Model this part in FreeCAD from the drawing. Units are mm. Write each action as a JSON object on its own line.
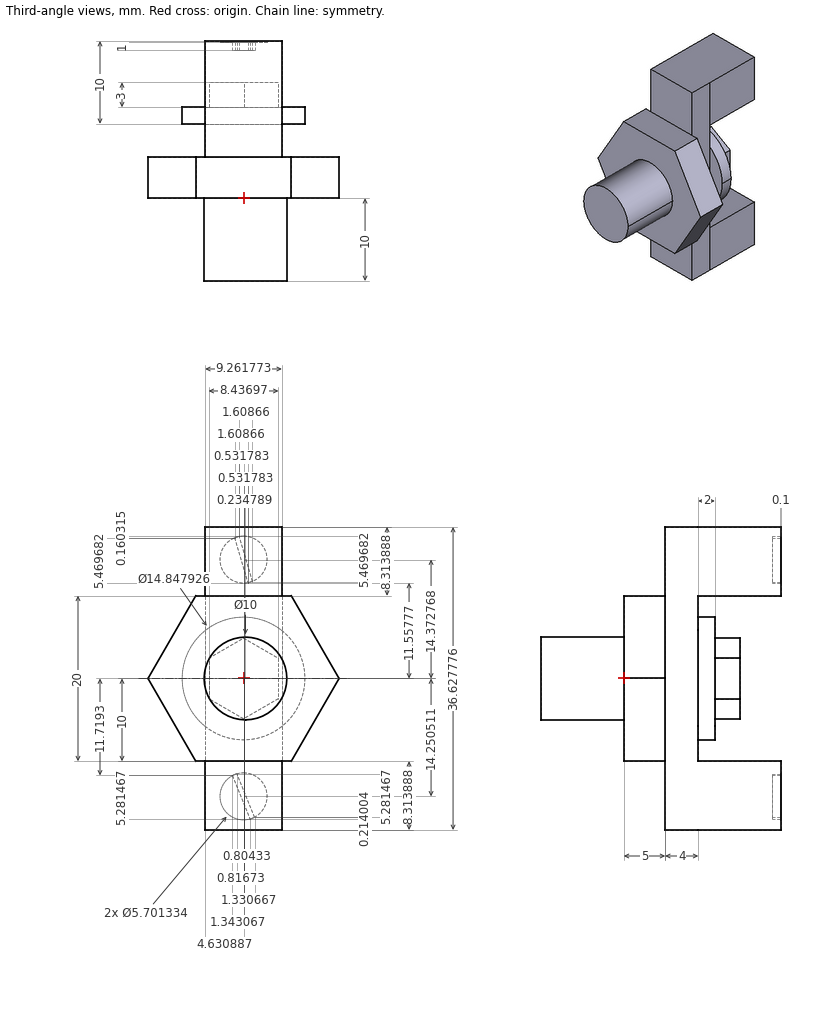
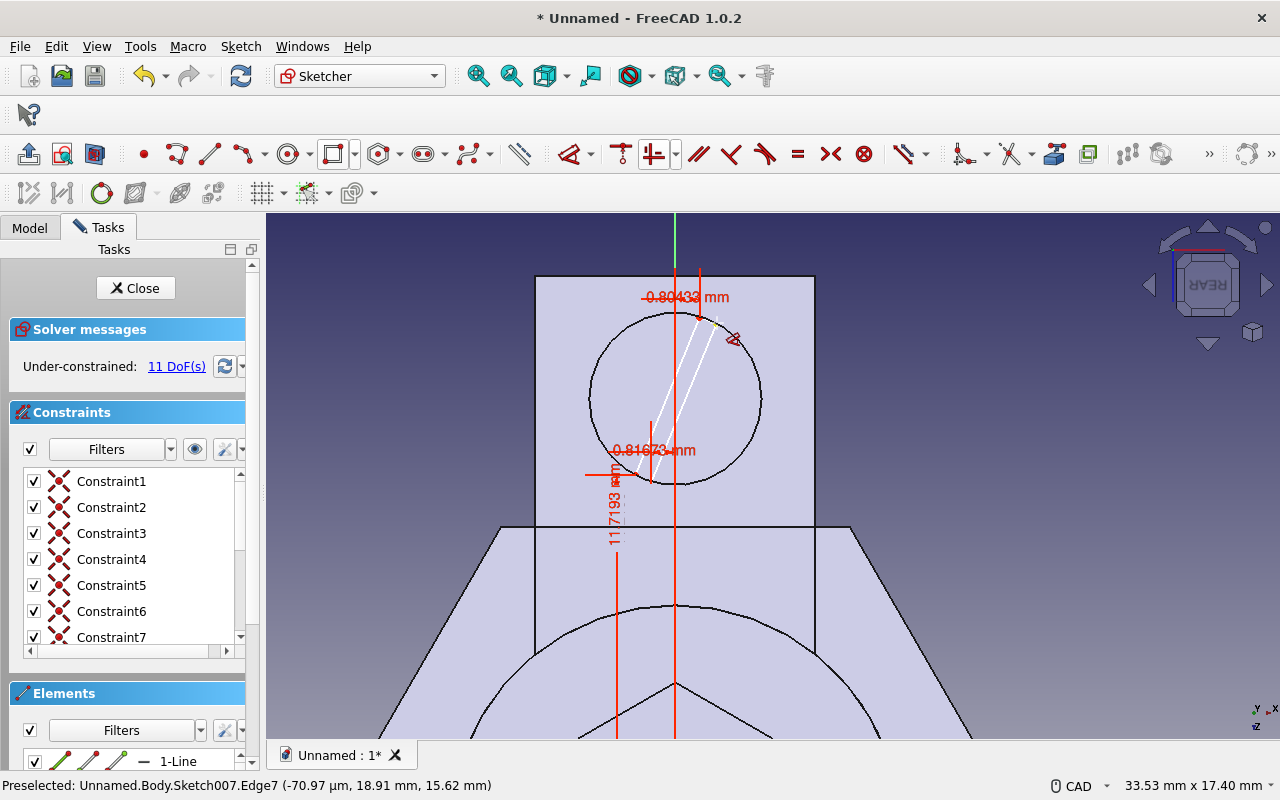
{"action": "left_click", "coordinate": [717, 324]}
{"action": "left_click", "coordinate": [696, 266]}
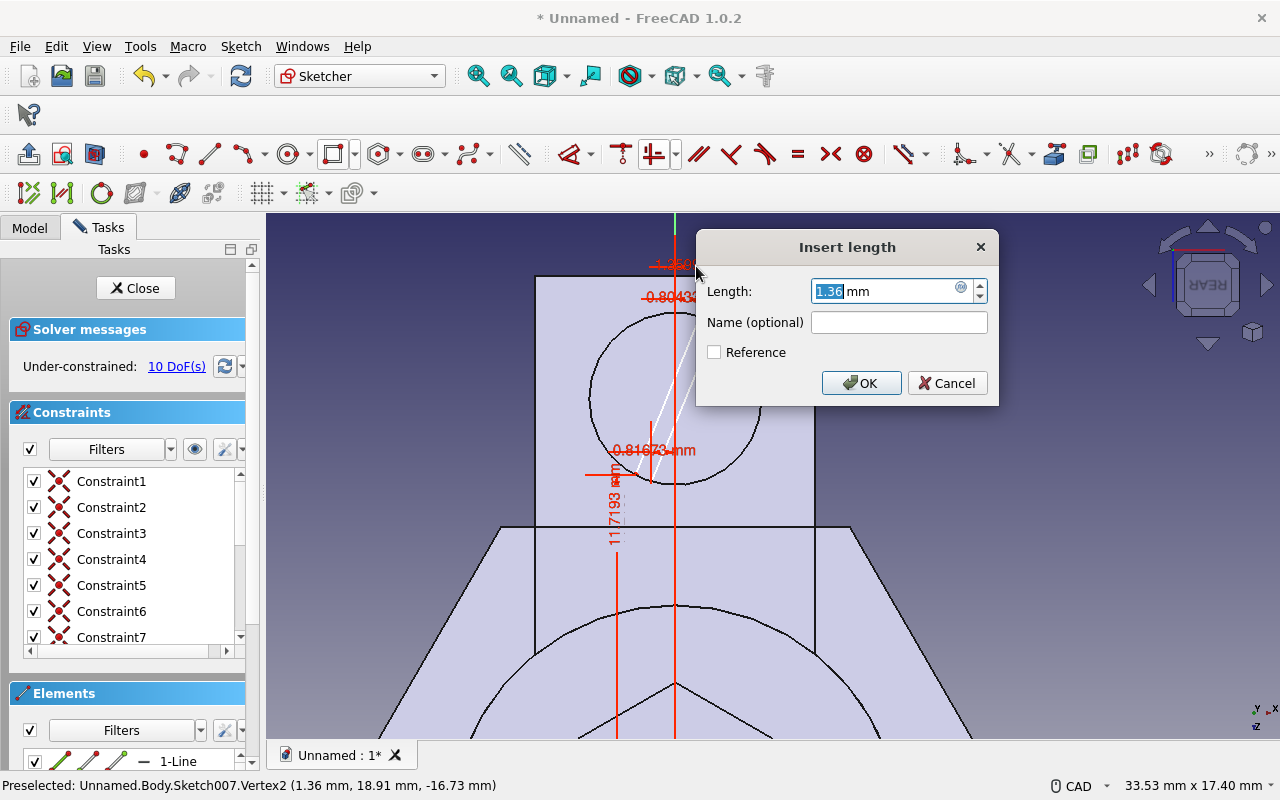
{"action": "type", "text": "1.330667"}
{"action": "key", "text": "Return"}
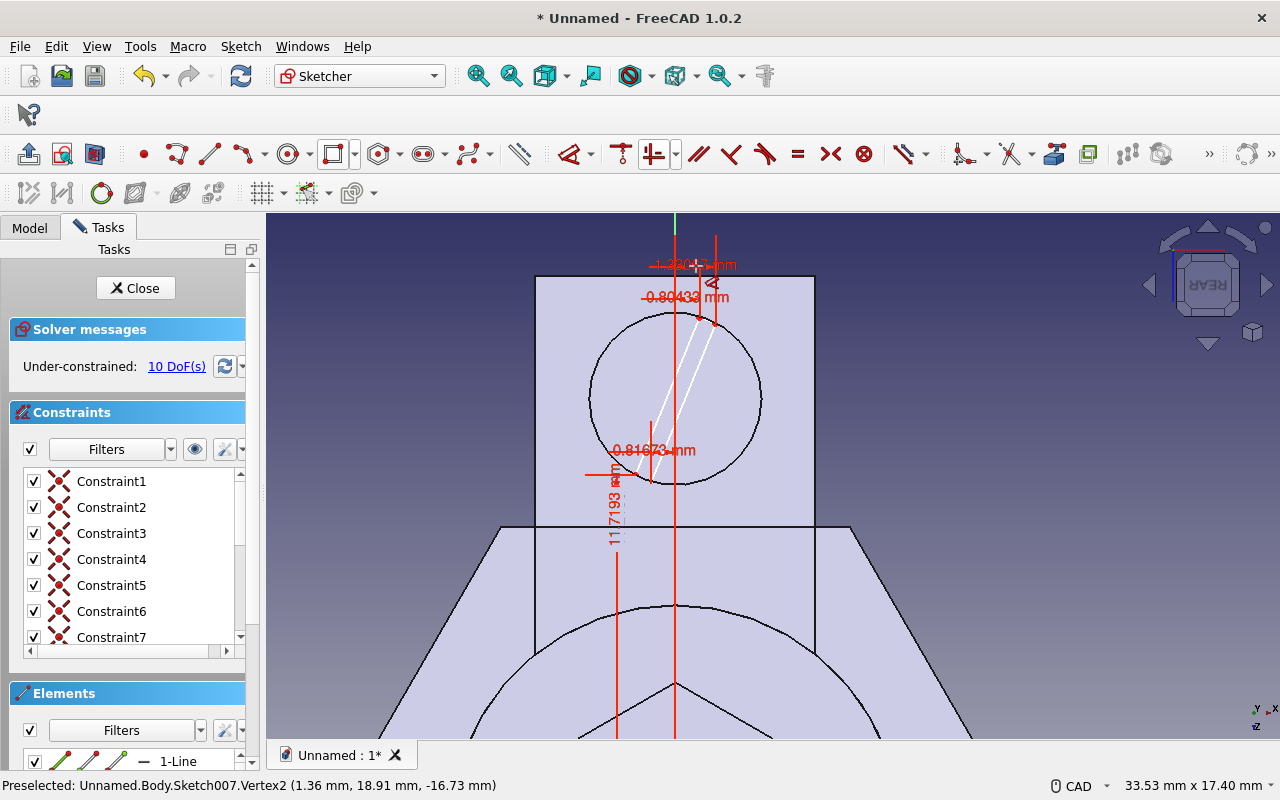
{"action": "left_click", "coordinate": [635, 475]}
{"action": "left_click", "coordinate": [641, 417]}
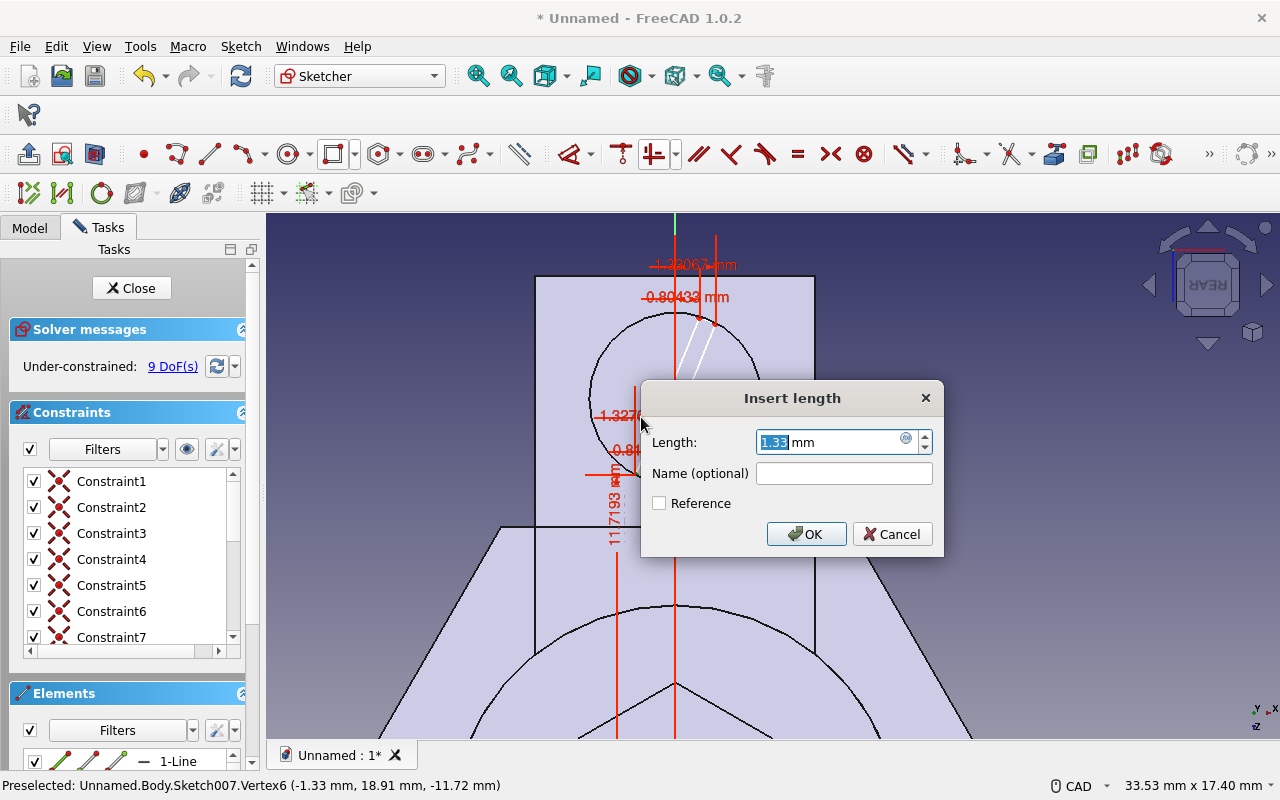
{"action": "type", "text": "1.343067"}
{"action": "key", "text": "Return"}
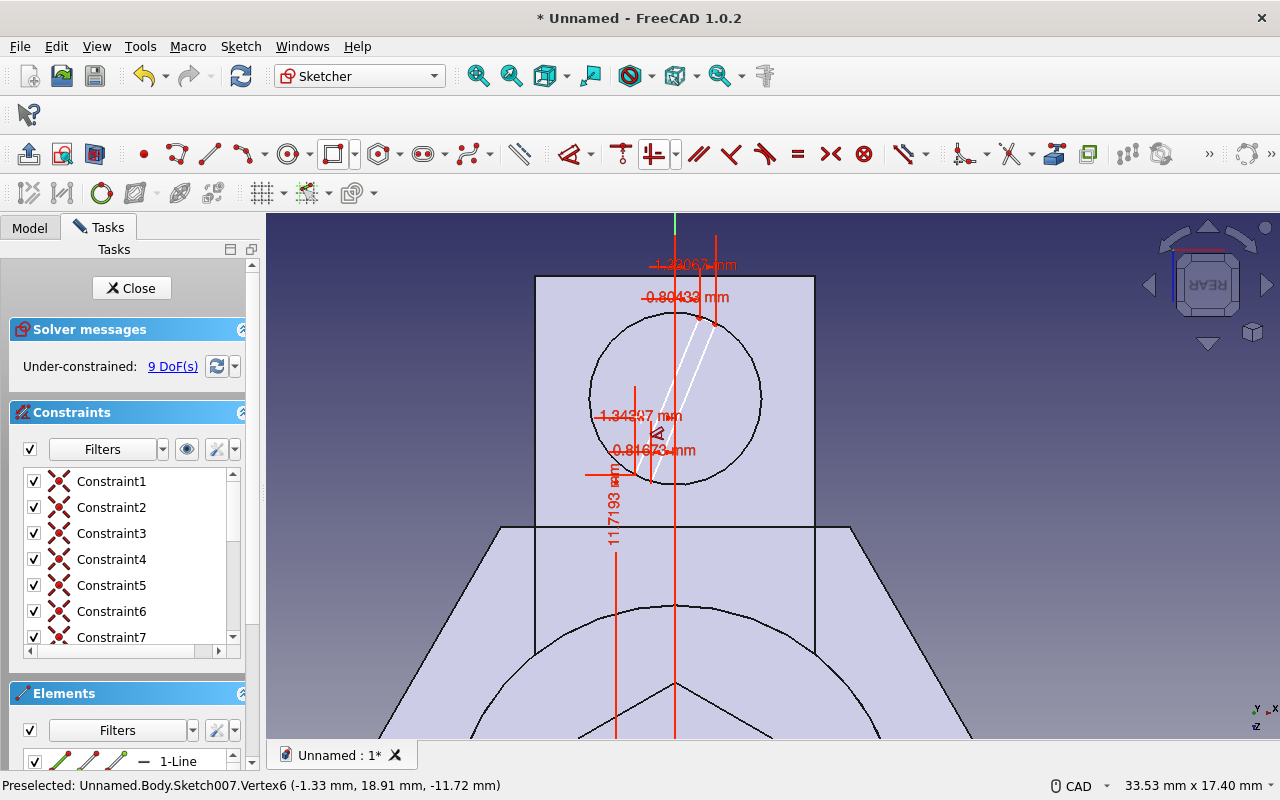
{"action": "scroll", "coordinate": [717, 322], "scroll_direction": "down", "scroll_amount": 6}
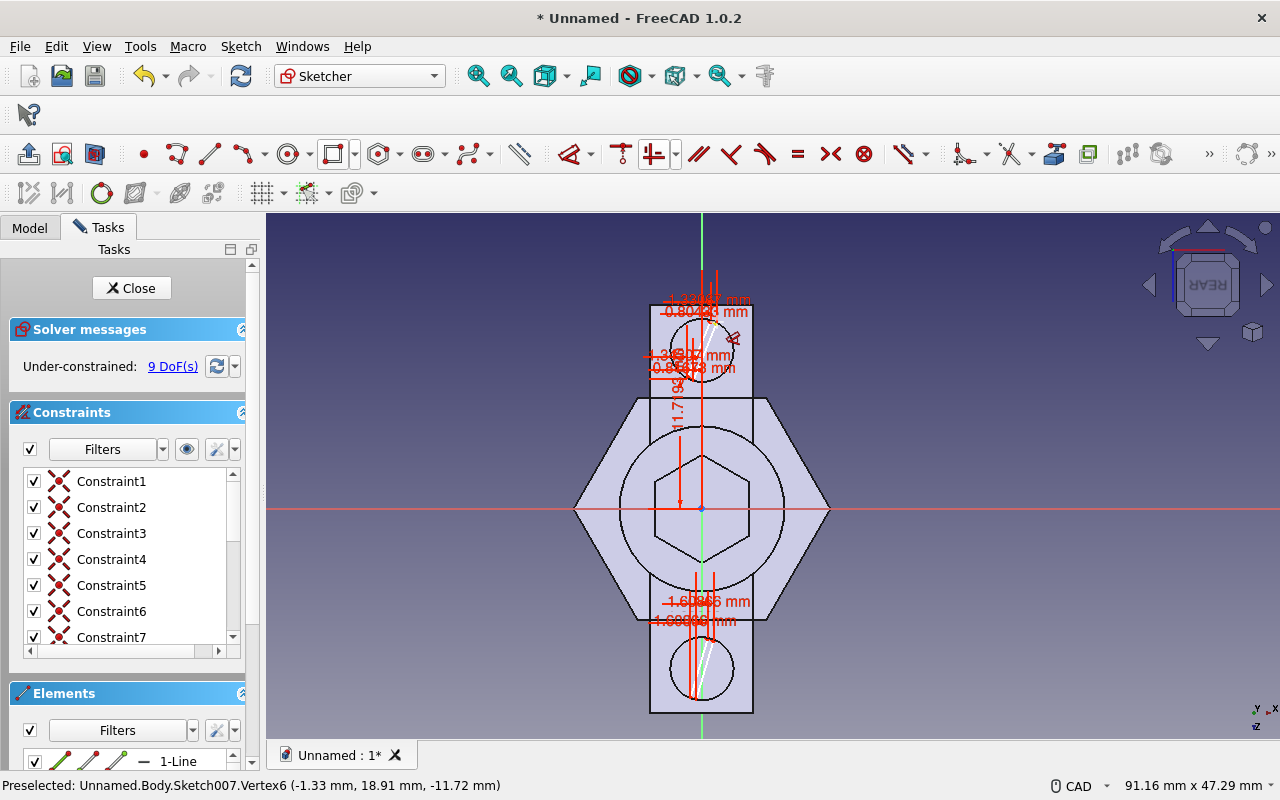
{"action": "scroll", "coordinate": [710, 581], "scroll_direction": "up", "scroll_amount": 11}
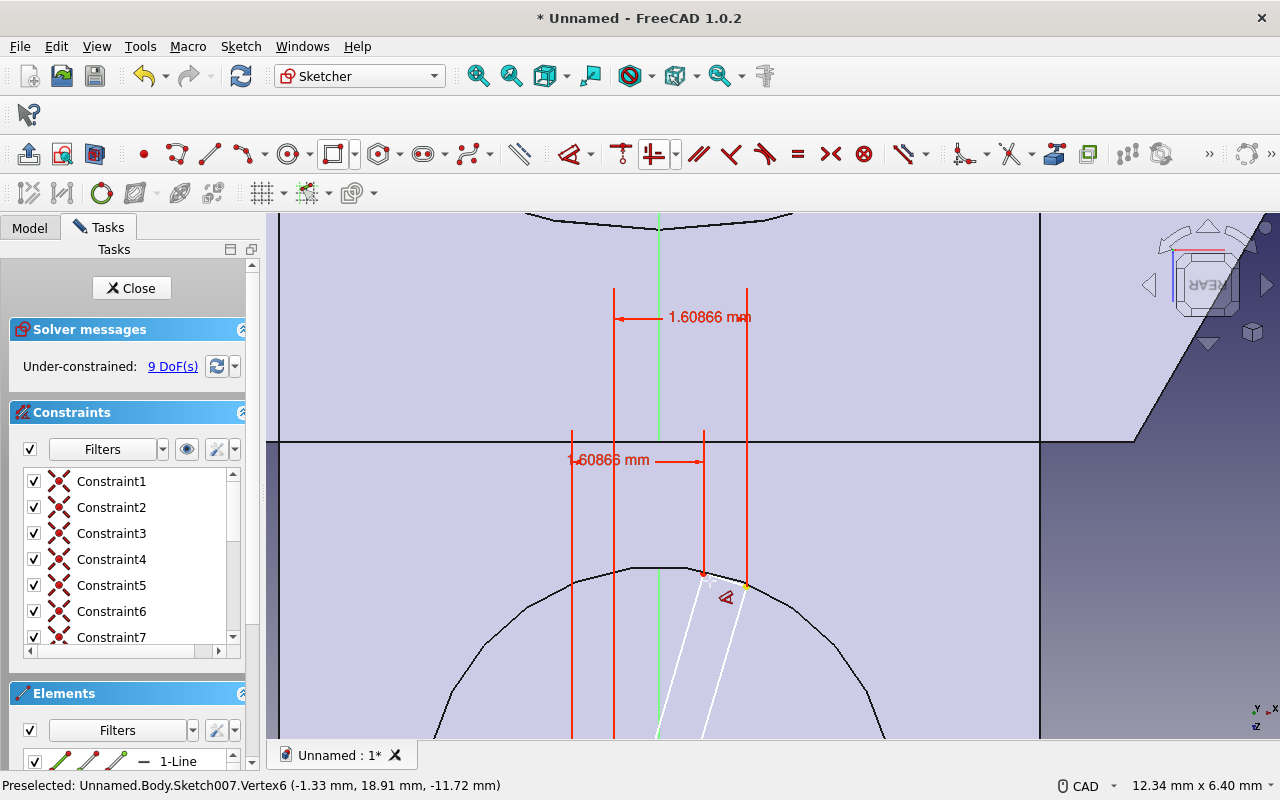
{"action": "left_click", "coordinate": [704, 573]}
{"action": "left_click", "coordinate": [697, 655]}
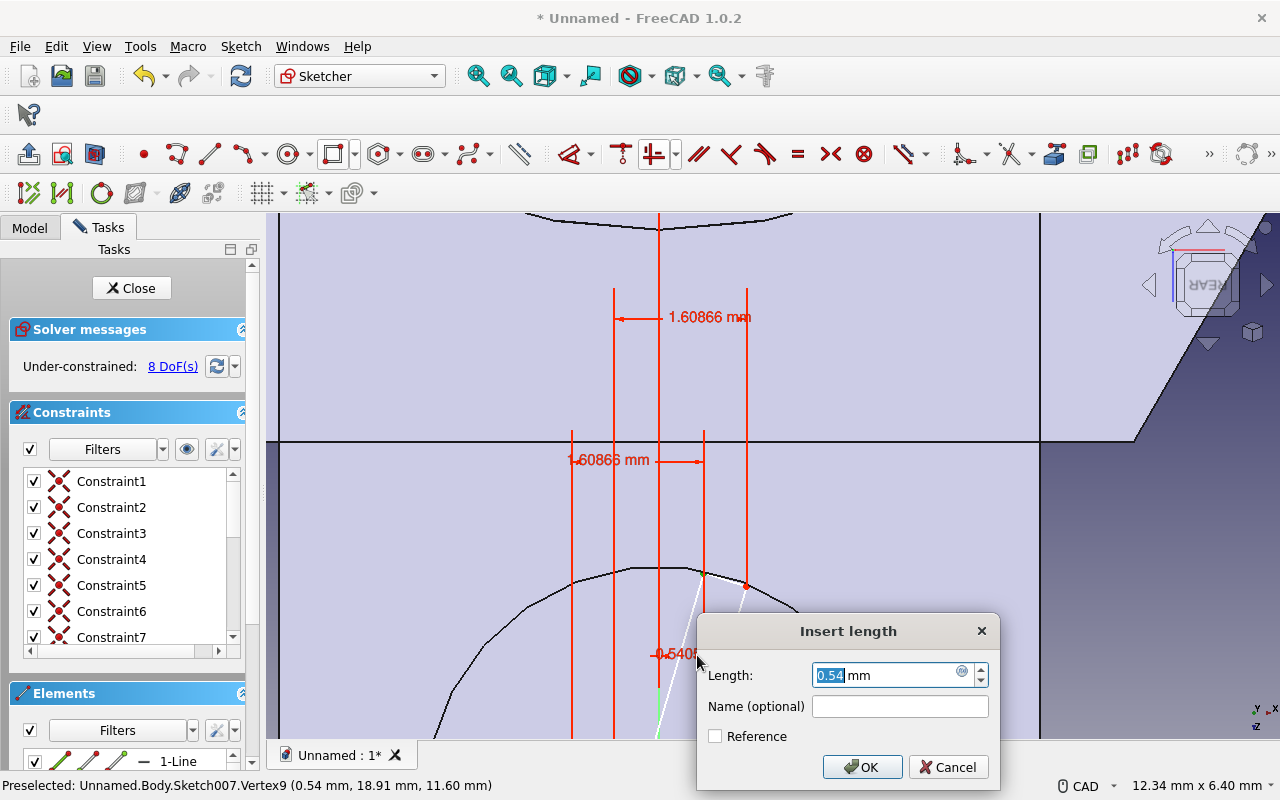
{"action": "type", "text": "0.531783"}
{"action": "key", "text": "Return"}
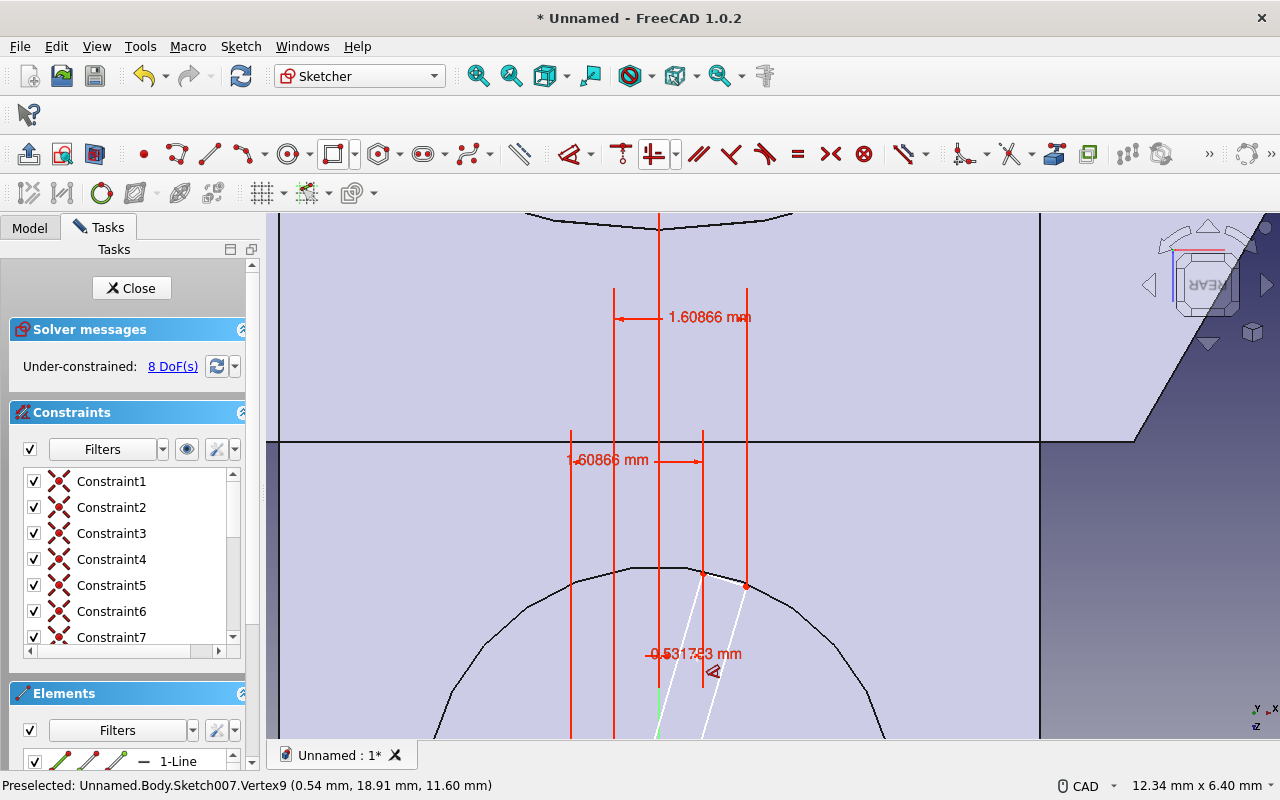
{"action": "scroll", "coordinate": [710, 582], "scroll_direction": "down", "scroll_amount": 11}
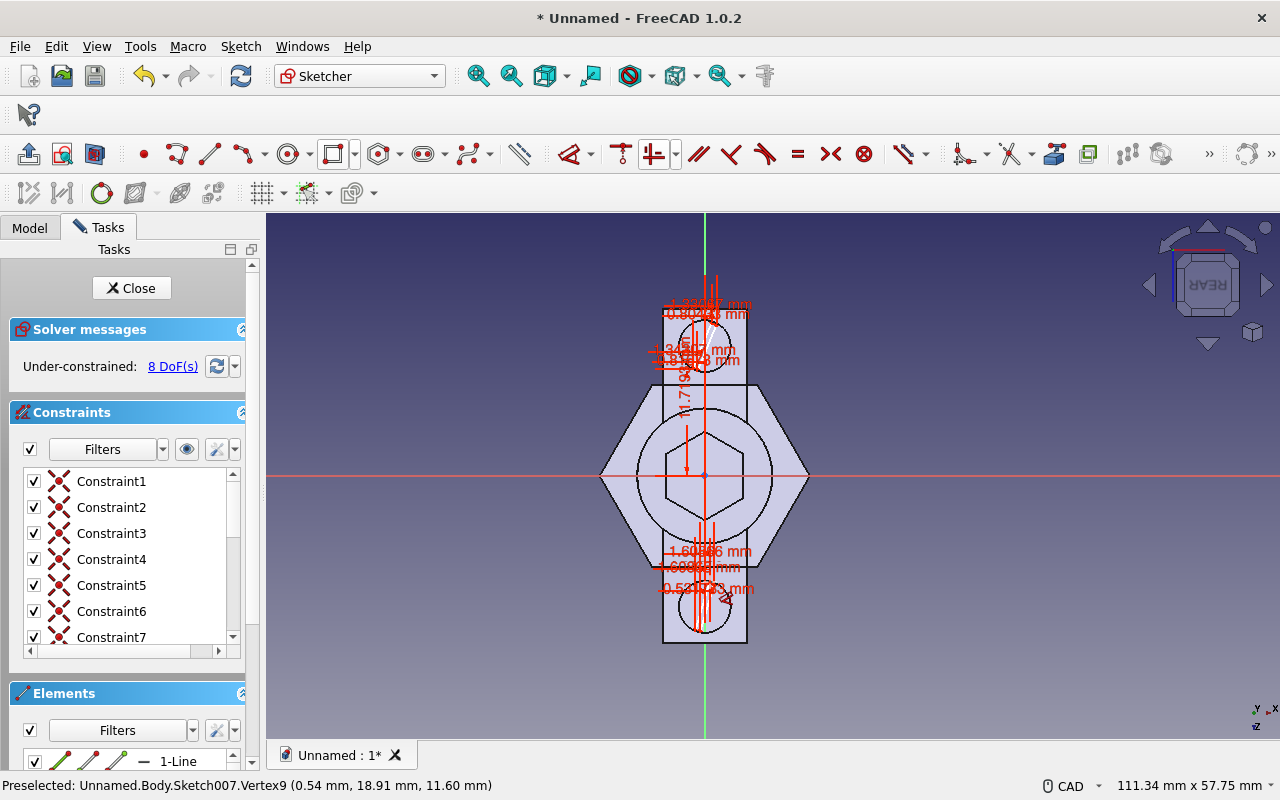
{"action": "scroll", "coordinate": [710, 582], "scroll_direction": "up", "scroll_amount": 5}